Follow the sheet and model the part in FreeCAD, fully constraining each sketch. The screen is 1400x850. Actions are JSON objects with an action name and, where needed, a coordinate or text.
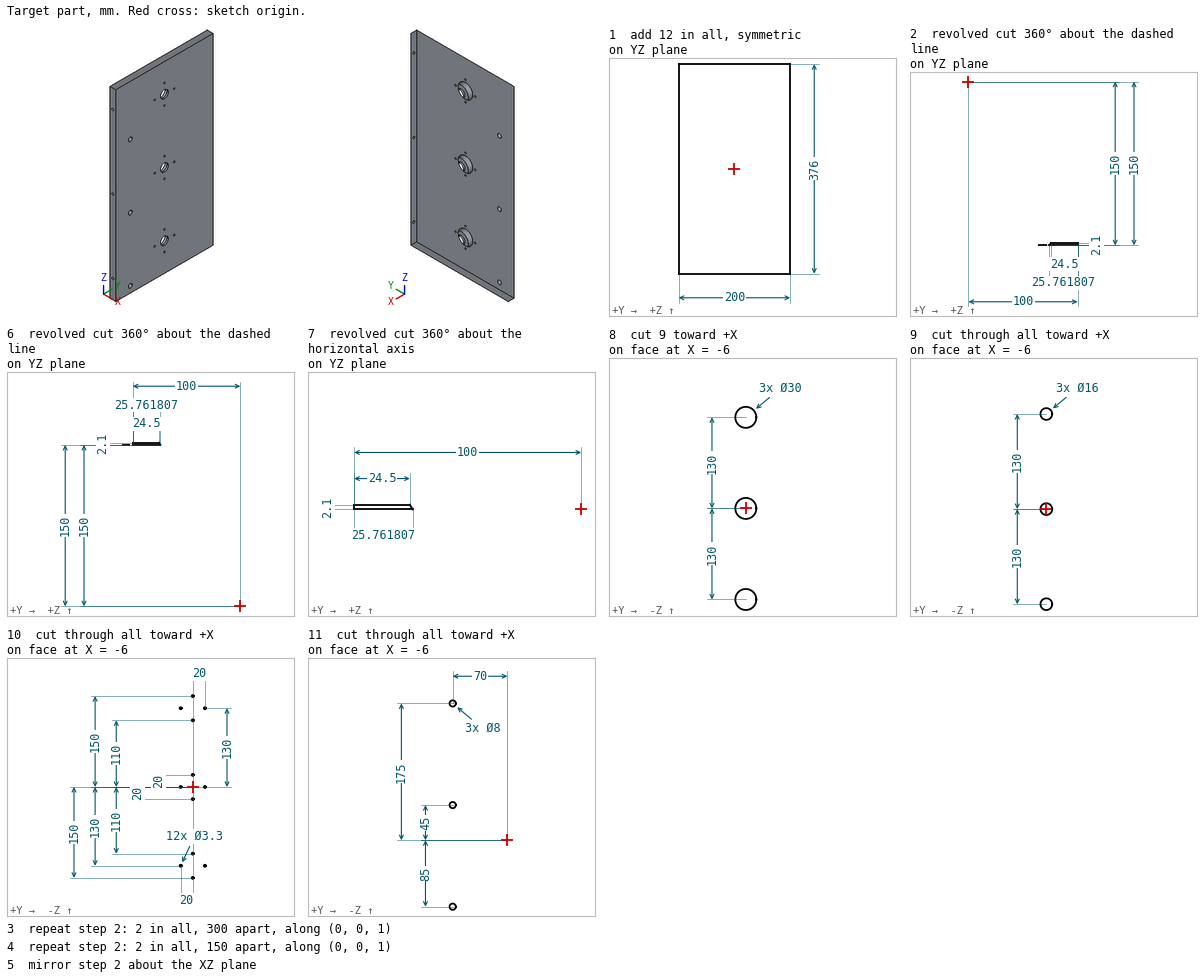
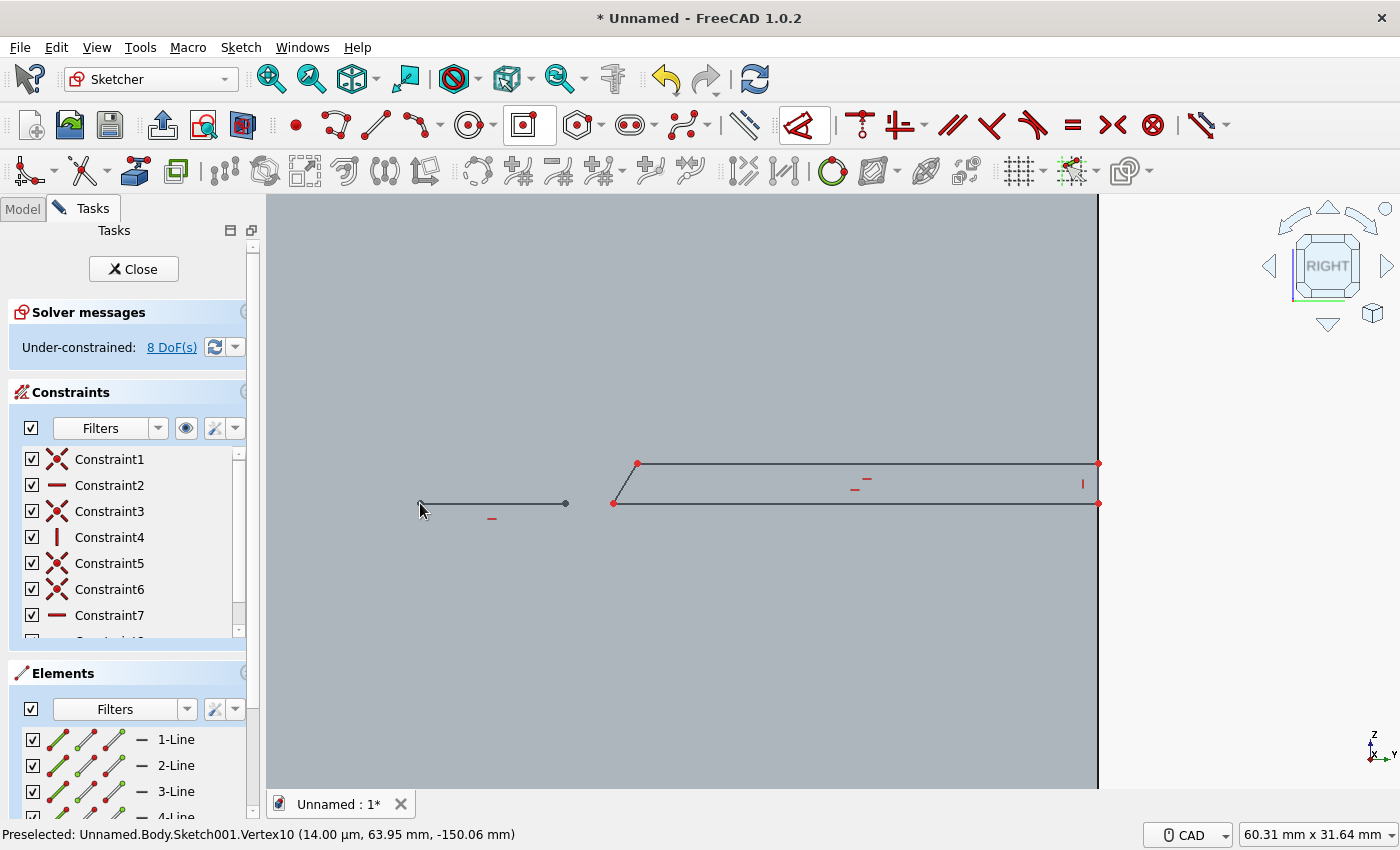
{"action": "left_click", "coordinate": [521, 504]}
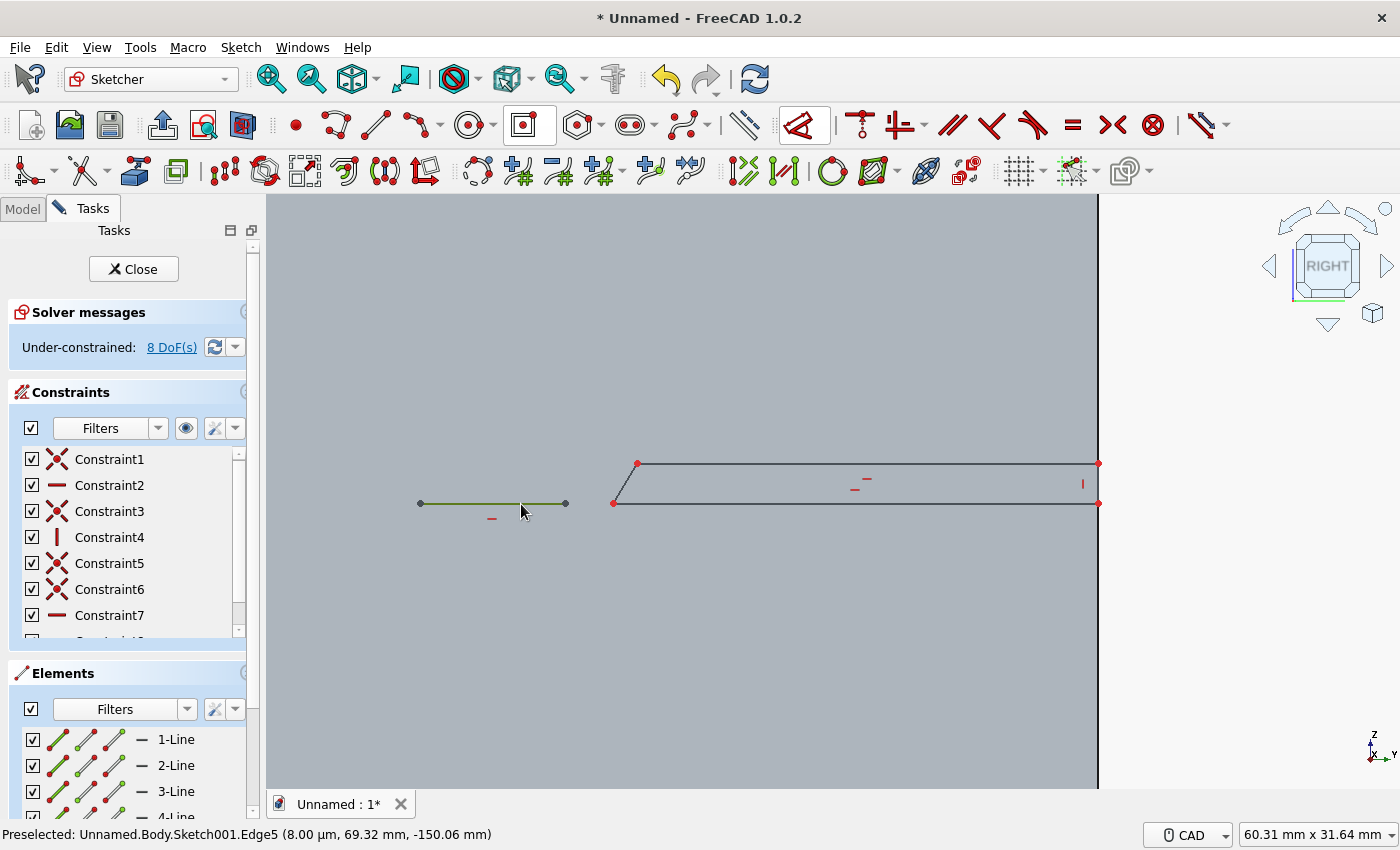
{"action": "left_click", "coordinate": [746, 126]}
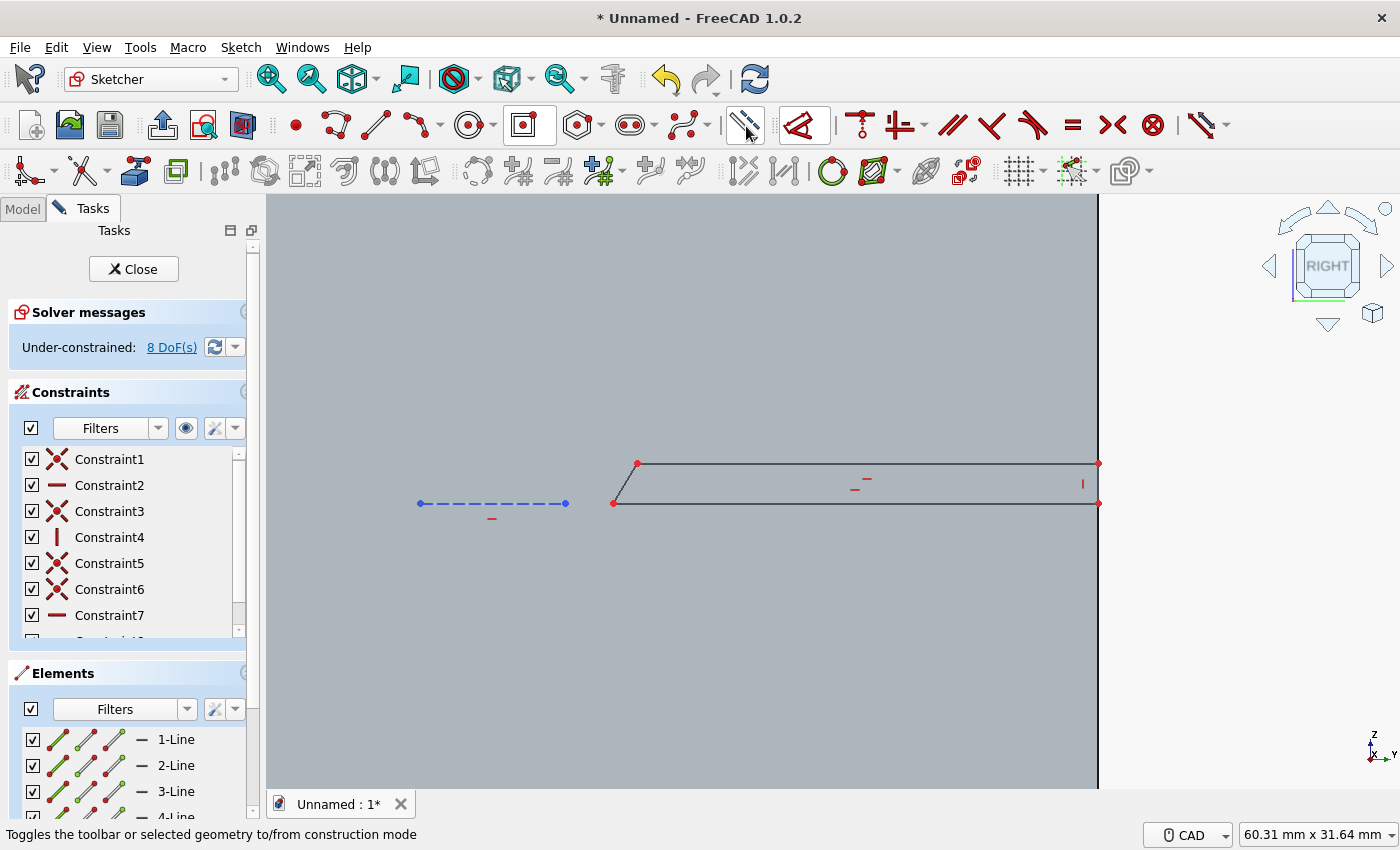
{"action": "left_click", "coordinate": [798, 126]}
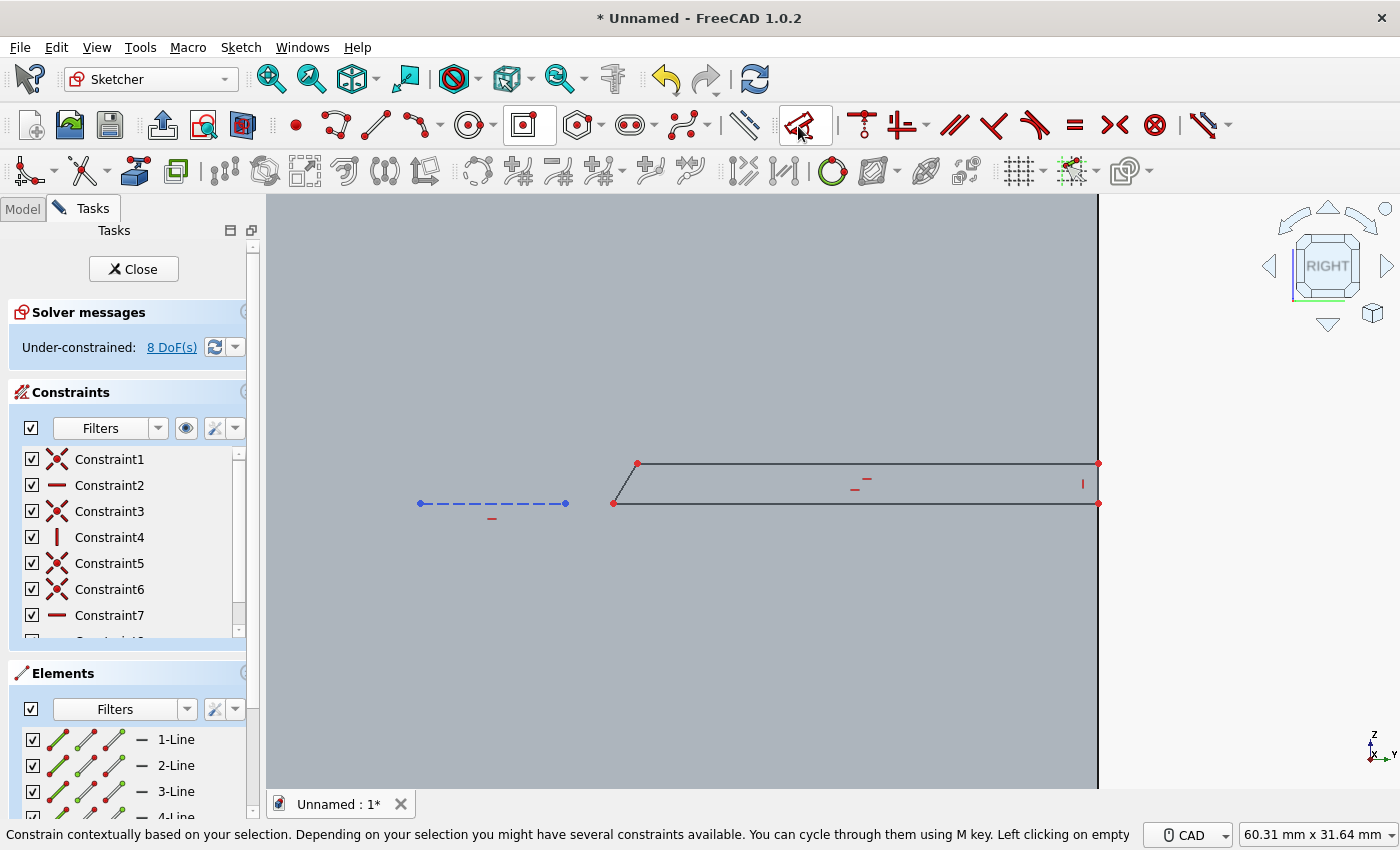
{"action": "left_click", "coordinate": [1098, 492]}
{"action": "left_click", "coordinate": [1132, 484]}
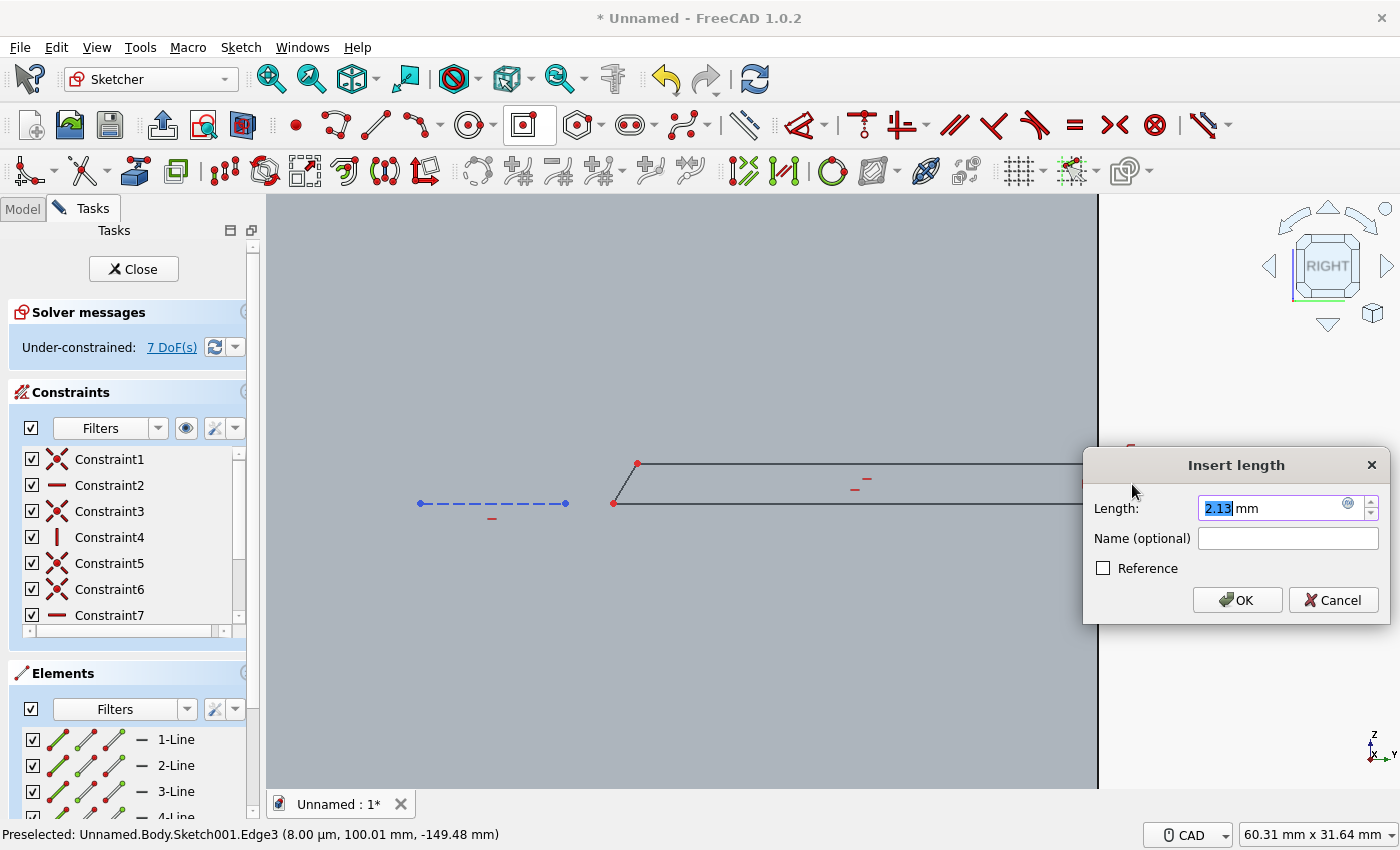
{"action": "type", "text": "2.1"}
{"action": "key", "text": "Return"}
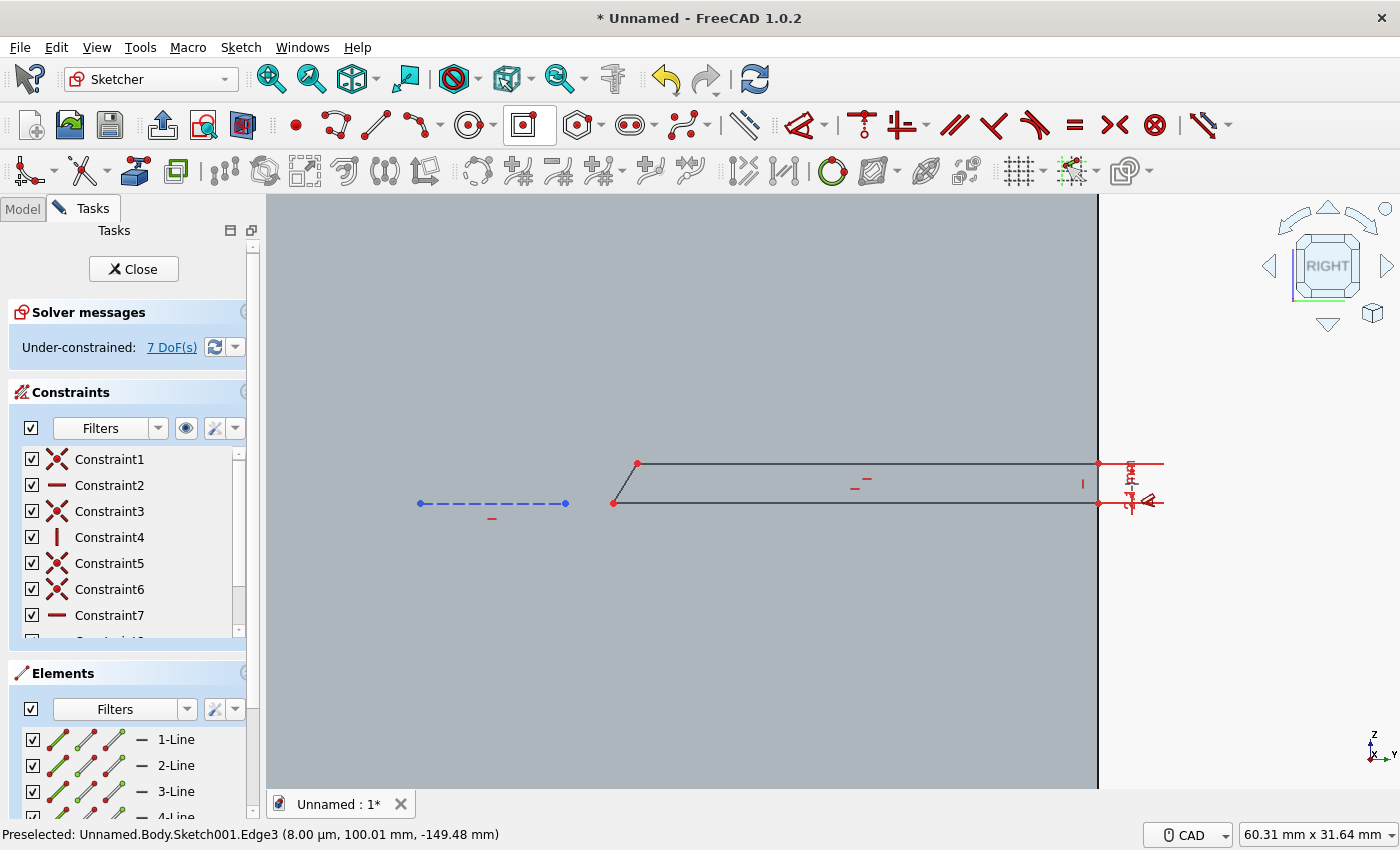
{"action": "left_click", "coordinate": [960, 464]}
{"action": "left_click", "coordinate": [867, 430]}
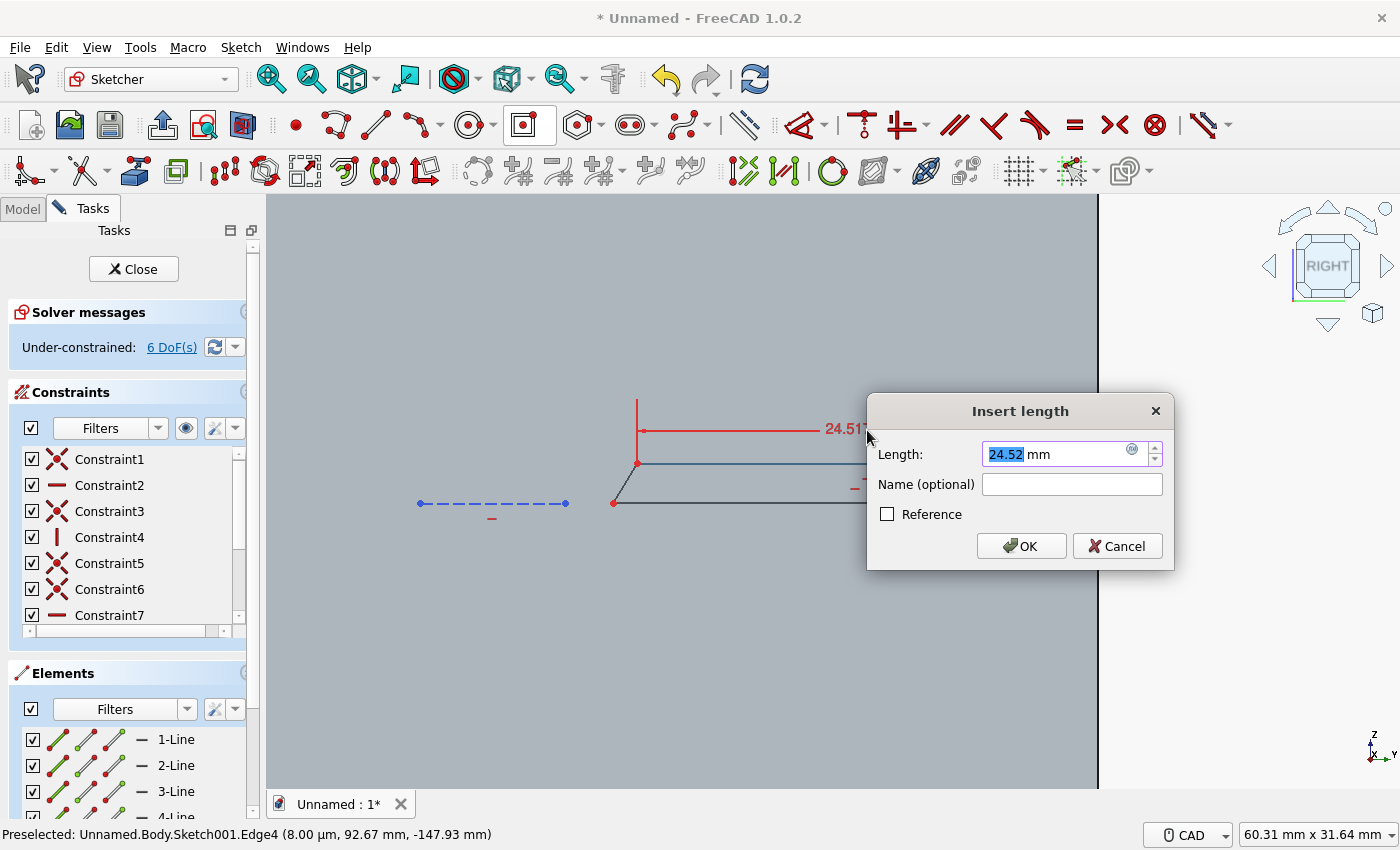
{"action": "type", "text": "24.5"}
{"action": "key", "text": "Return"}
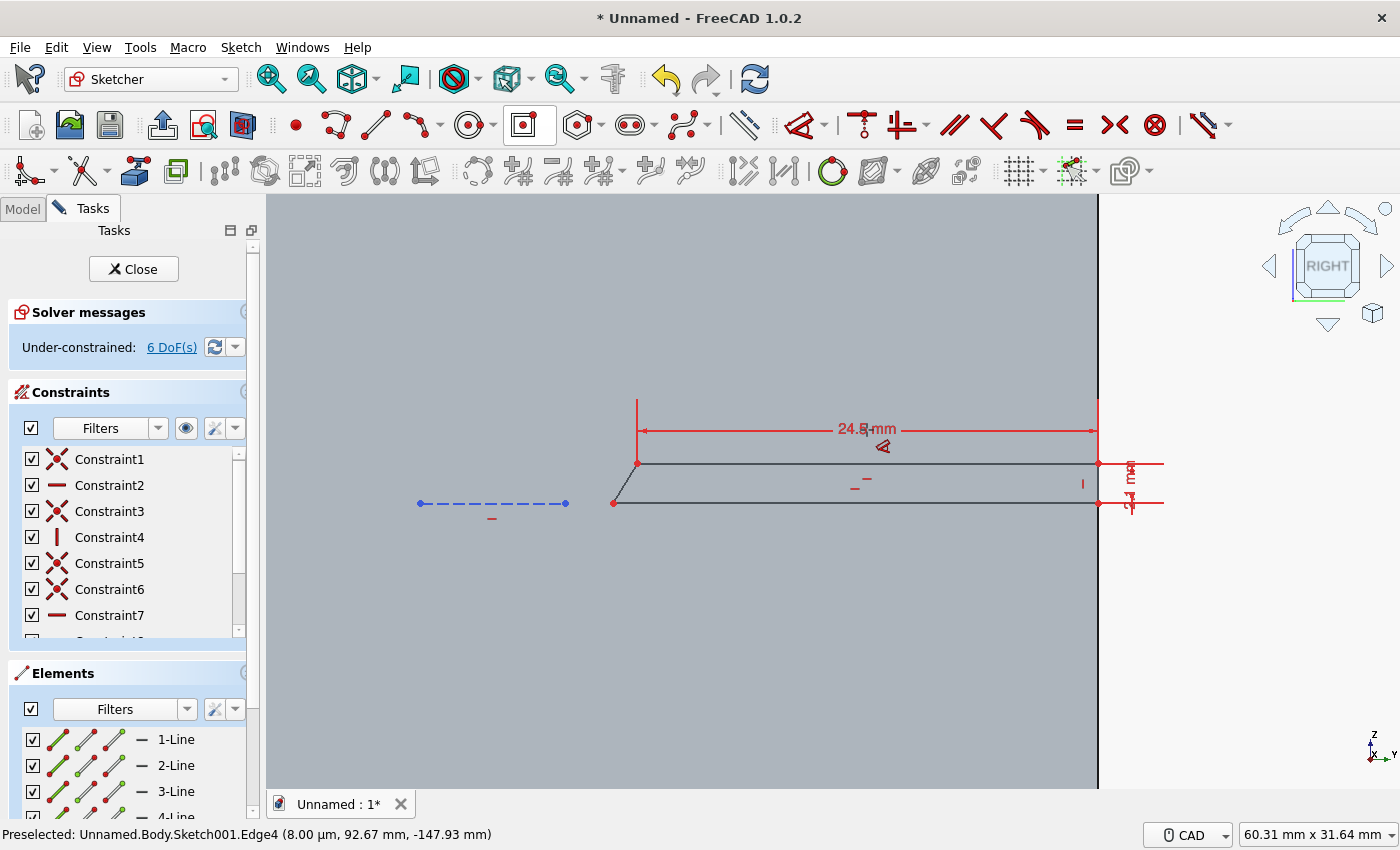
{"action": "left_click", "coordinate": [613, 503]}
{"action": "left_click", "coordinate": [647, 363]}